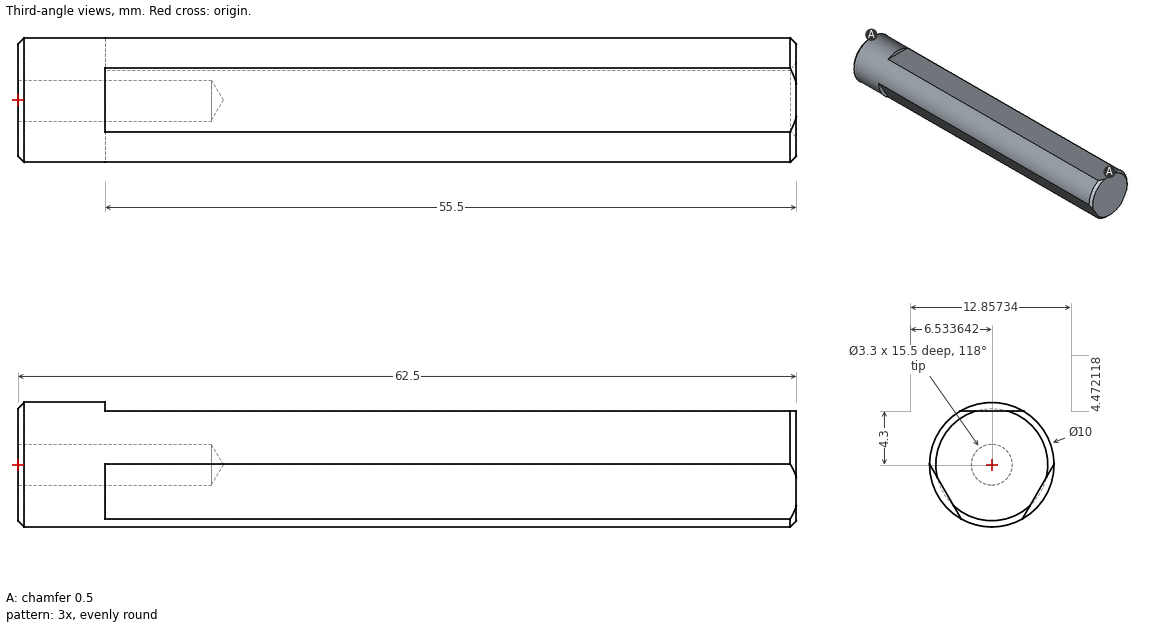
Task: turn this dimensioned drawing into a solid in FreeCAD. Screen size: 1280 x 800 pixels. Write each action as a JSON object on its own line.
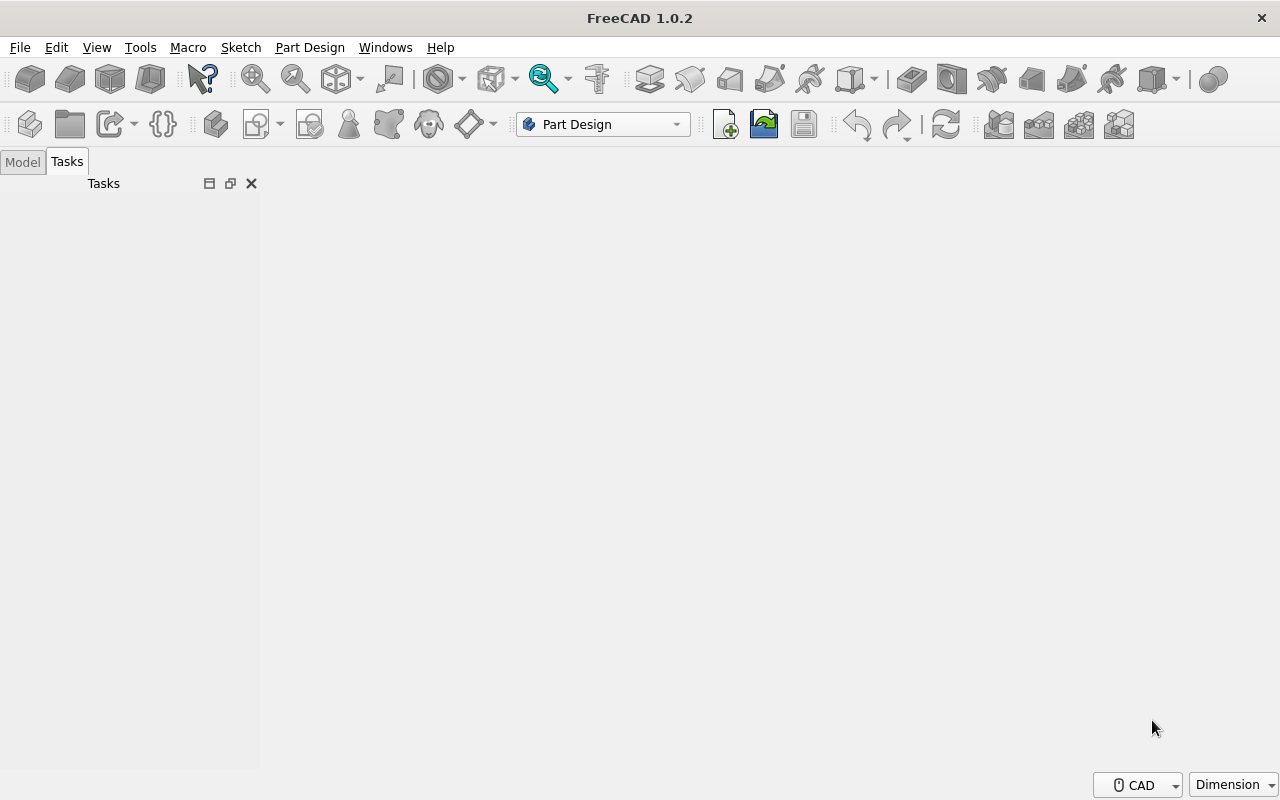
{"action": "left_click", "coordinate": [724, 124]}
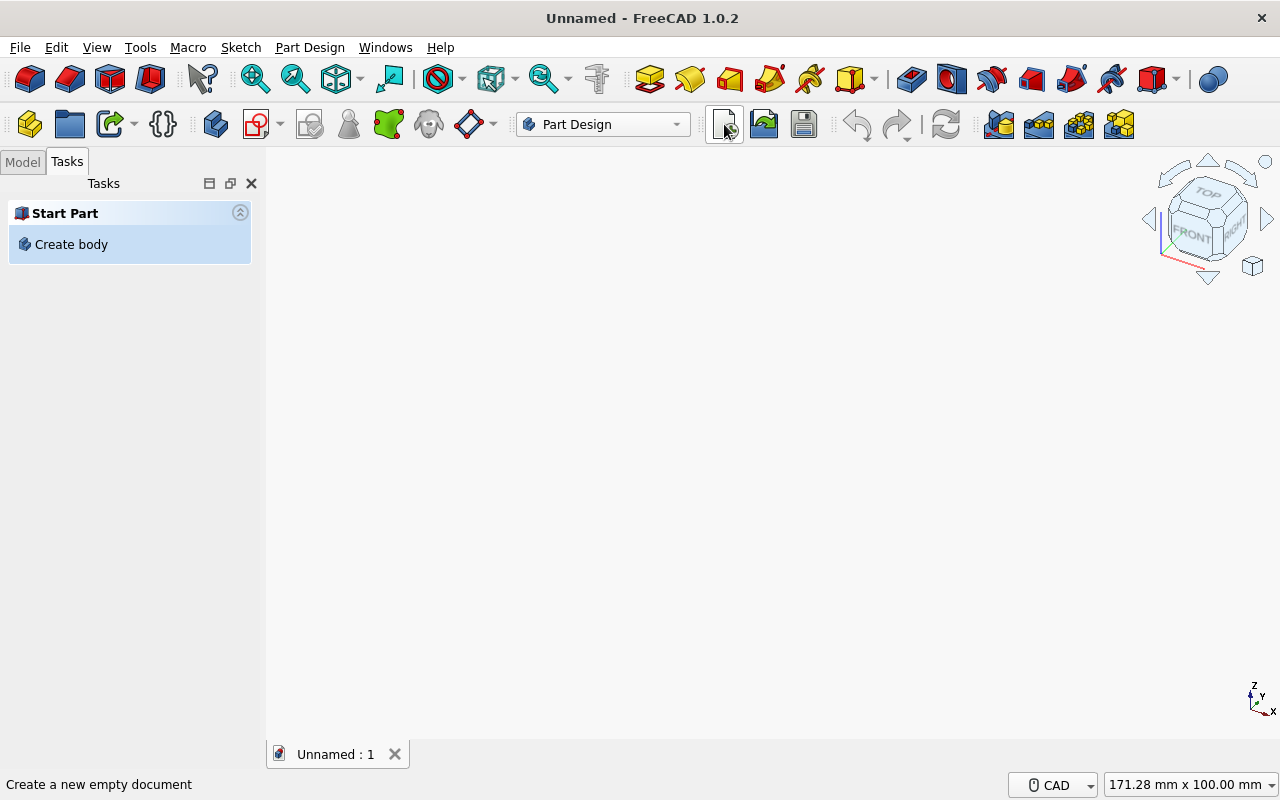
{"action": "left_click", "coordinate": [256, 124]}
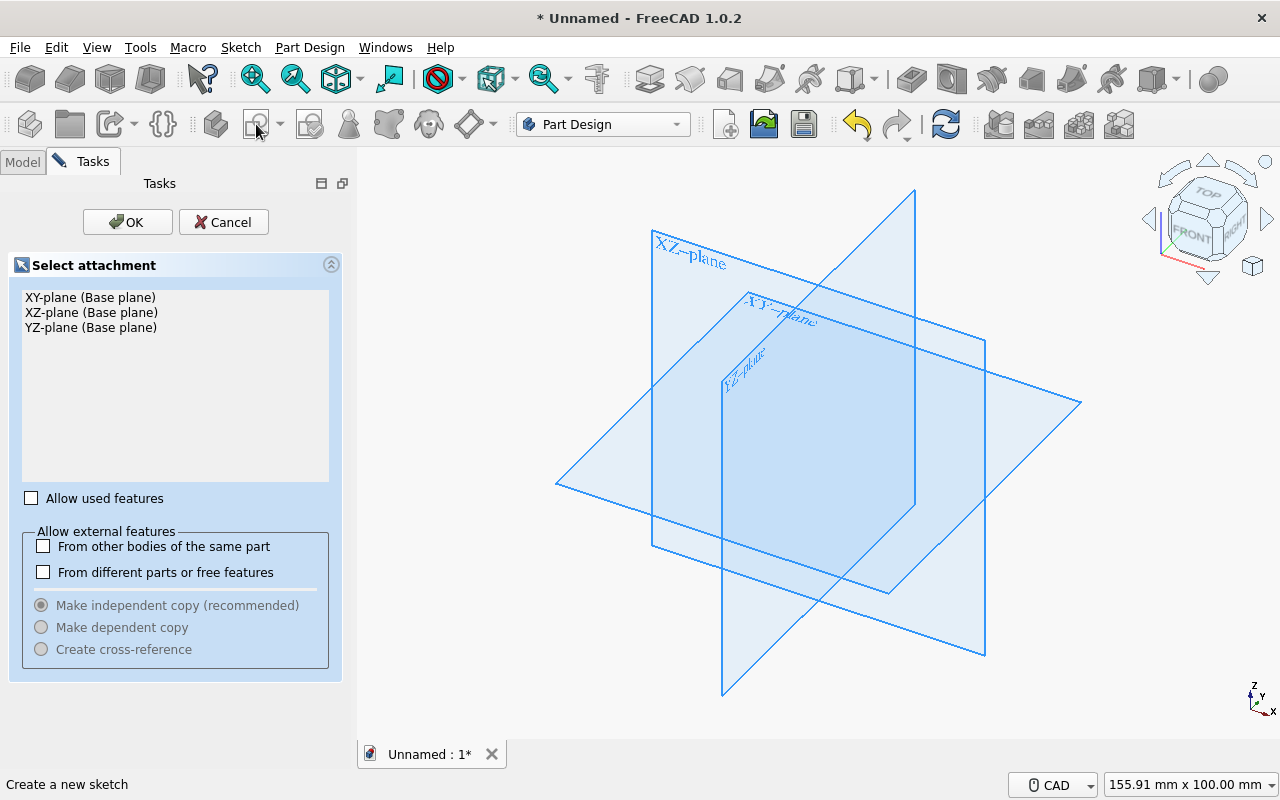
{"action": "left_click", "coordinate": [82, 328]}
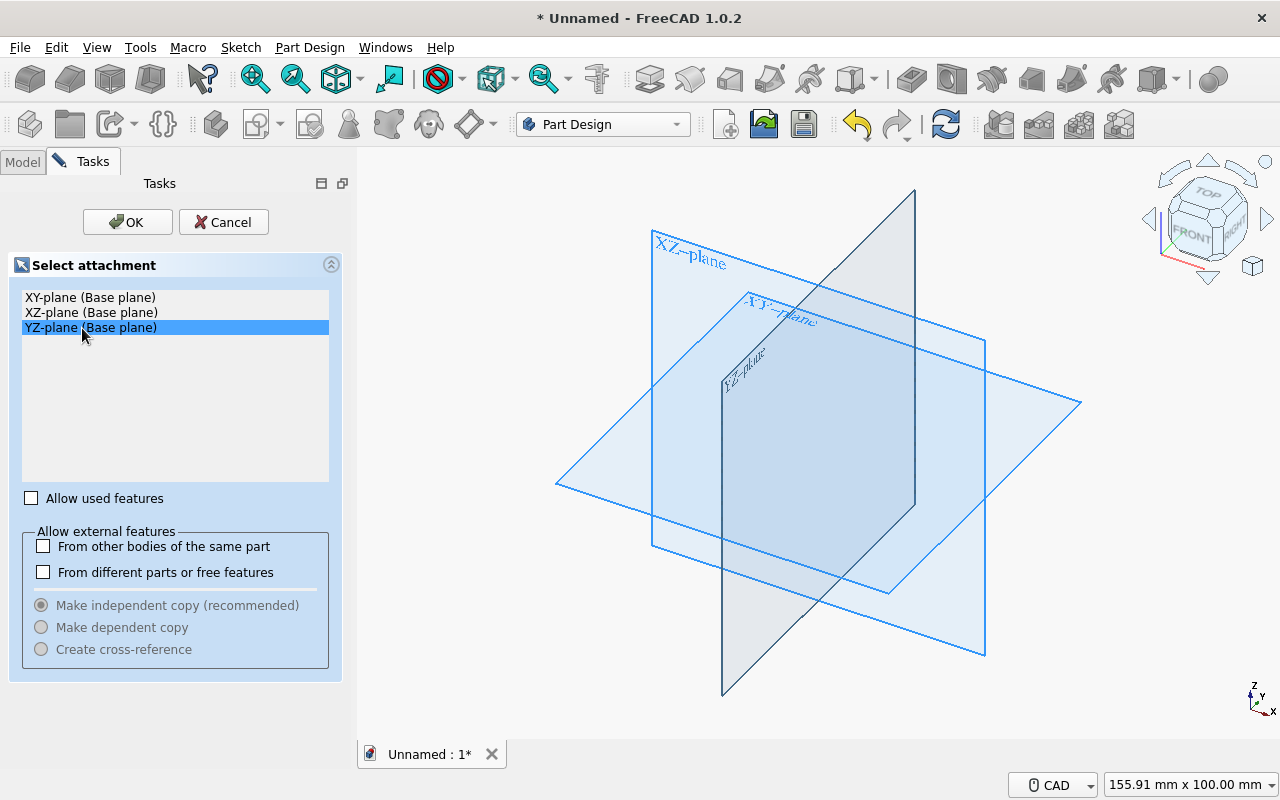
{"action": "left_click", "coordinate": [128, 222]}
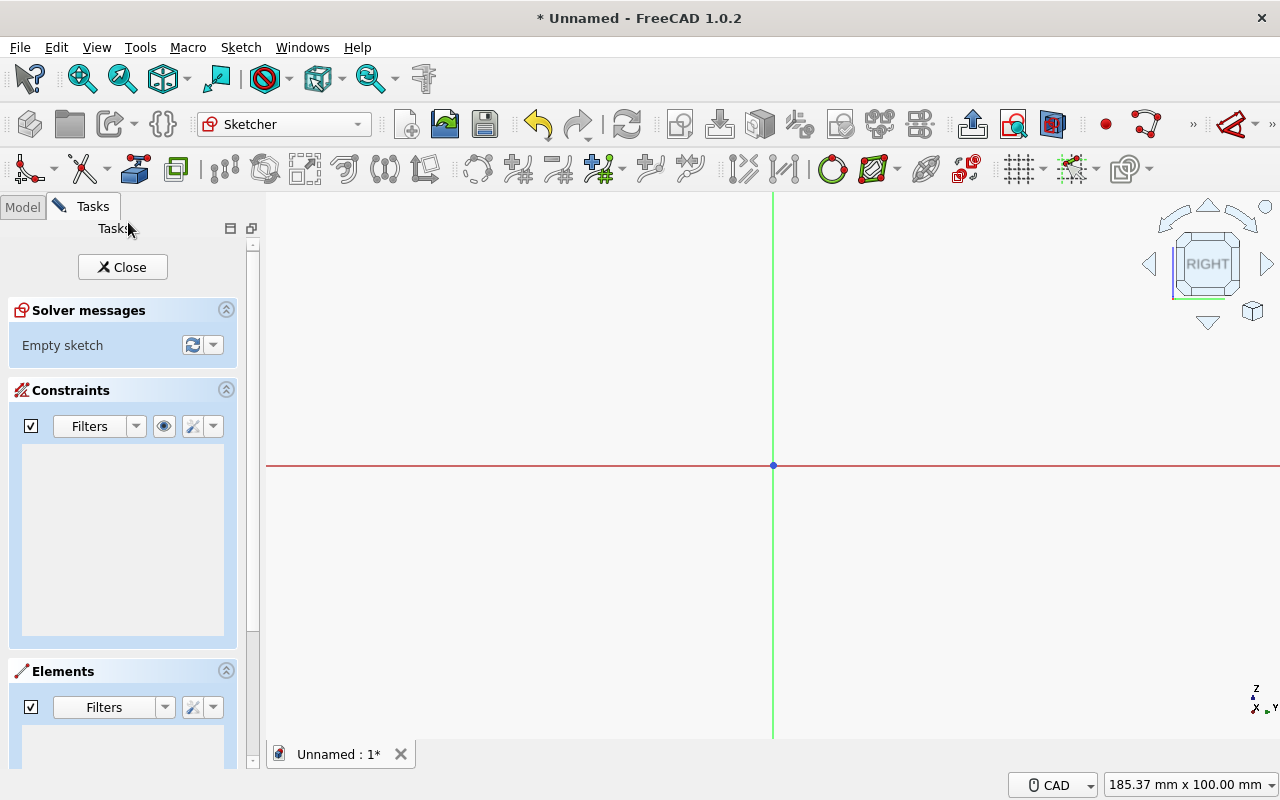
{"action": "scroll", "coordinate": [787, 465], "scroll_direction": "up", "scroll_amount": 9}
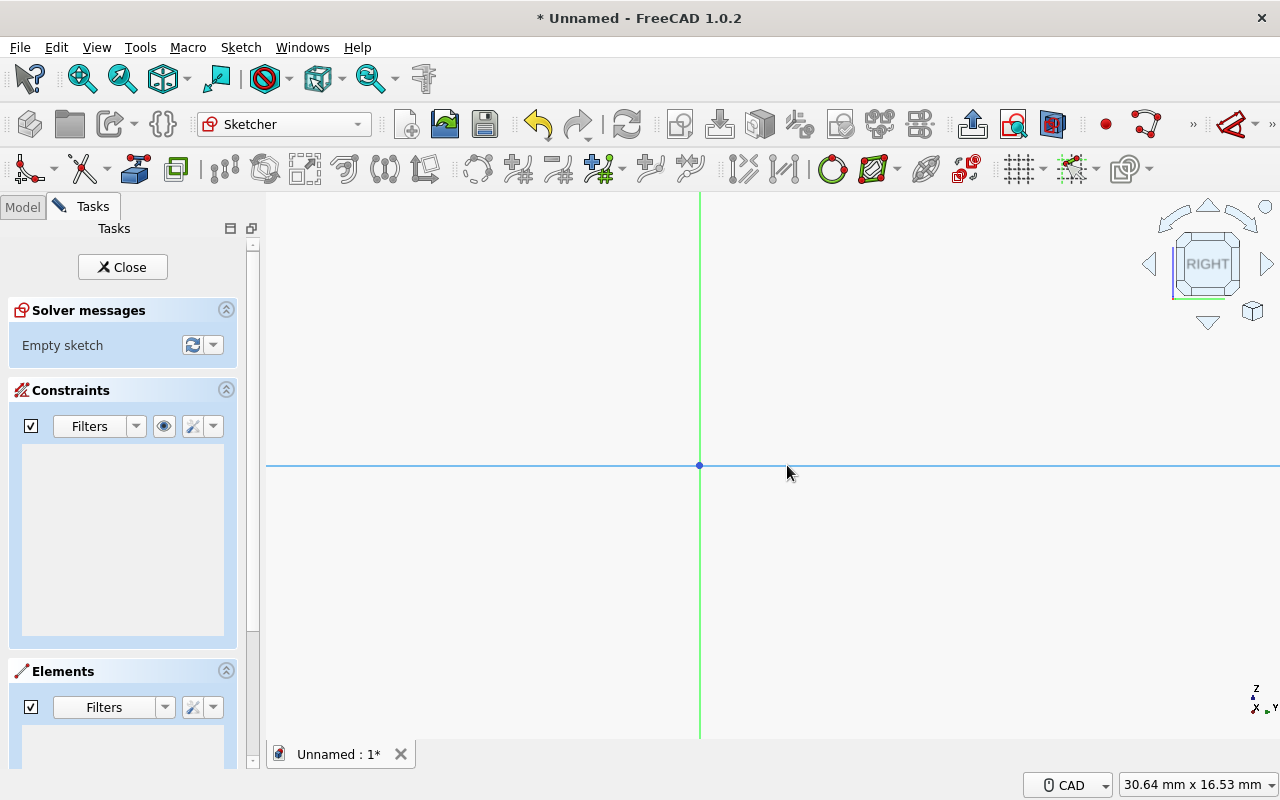
{"action": "key", "text": "g c"}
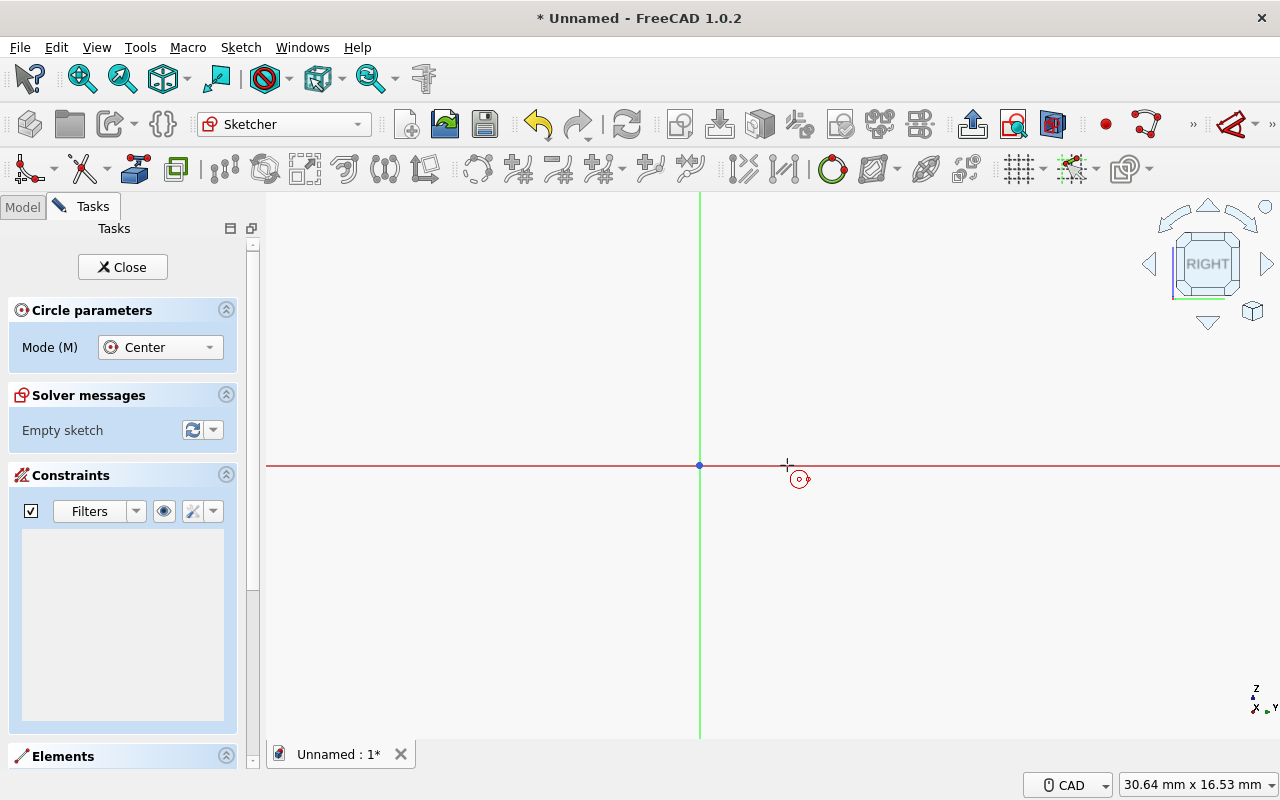
{"action": "left_click", "coordinate": [700, 466]}
{"action": "mouse_move", "coordinate": [817, 349]}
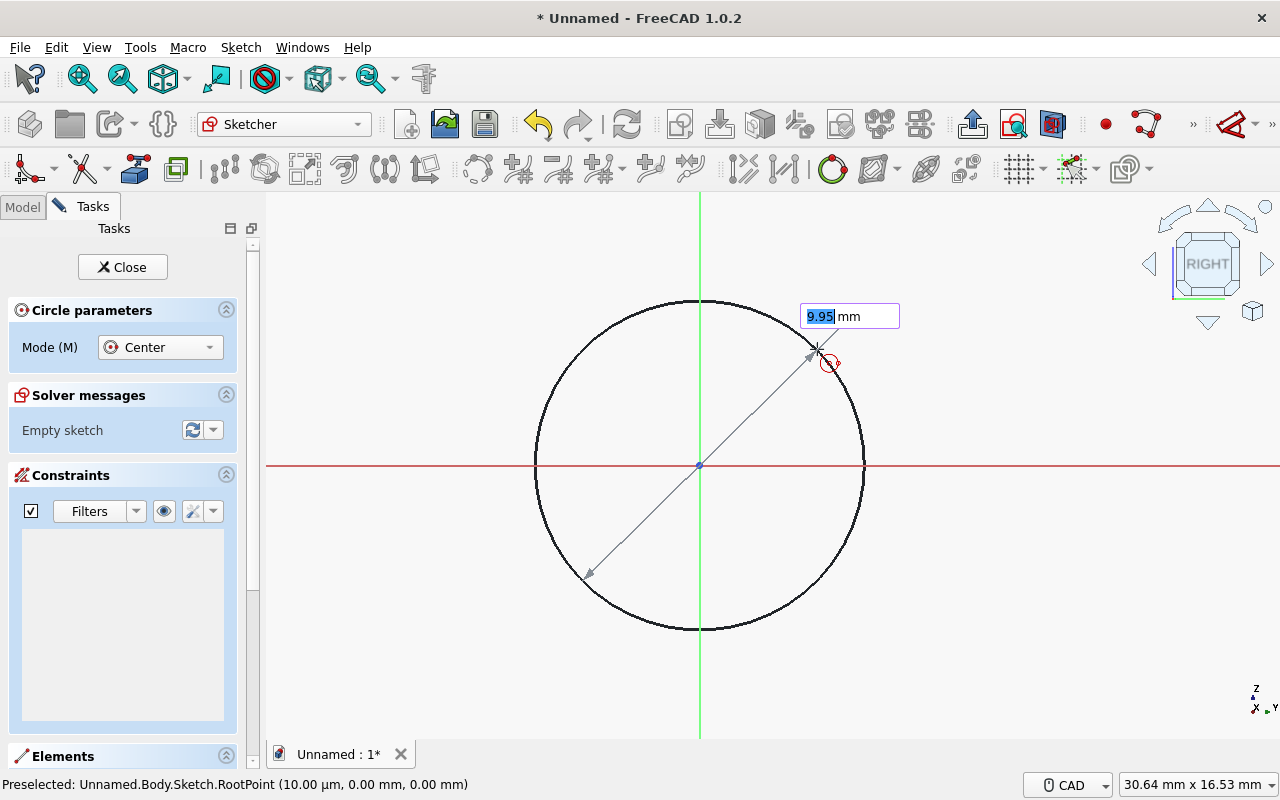
{"action": "type", "text": "10"}
{"action": "key", "text": "Return"}
{"action": "key", "text": "Escape"}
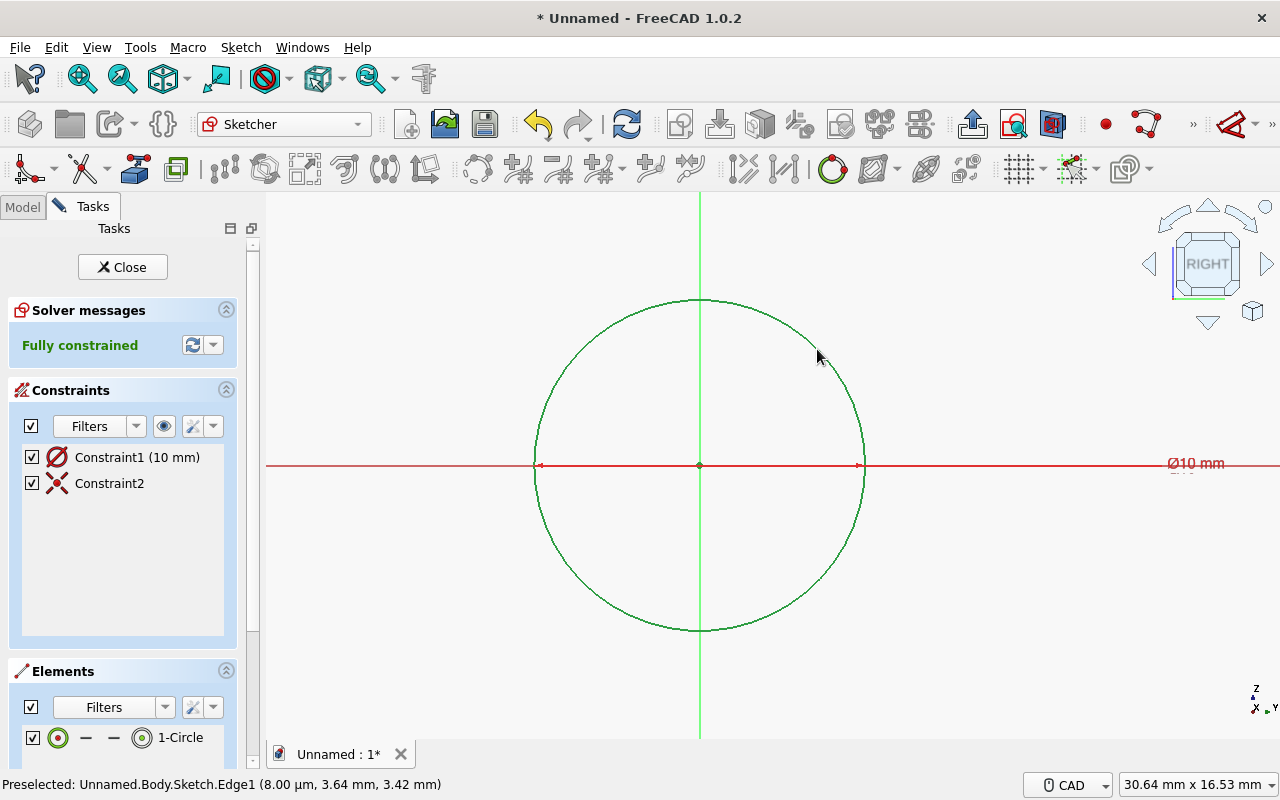
{"action": "left_click", "coordinate": [123, 267]}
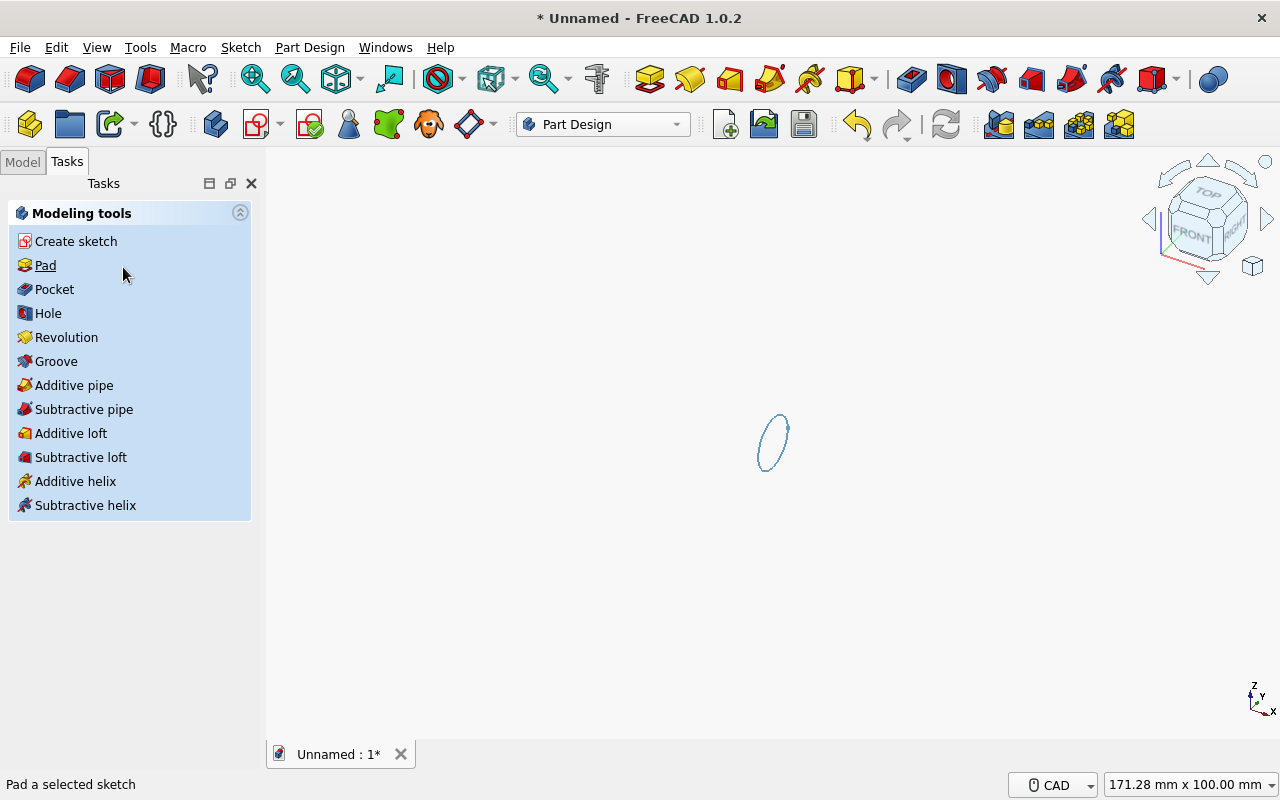
{"action": "left_click", "coordinate": [650, 80]}